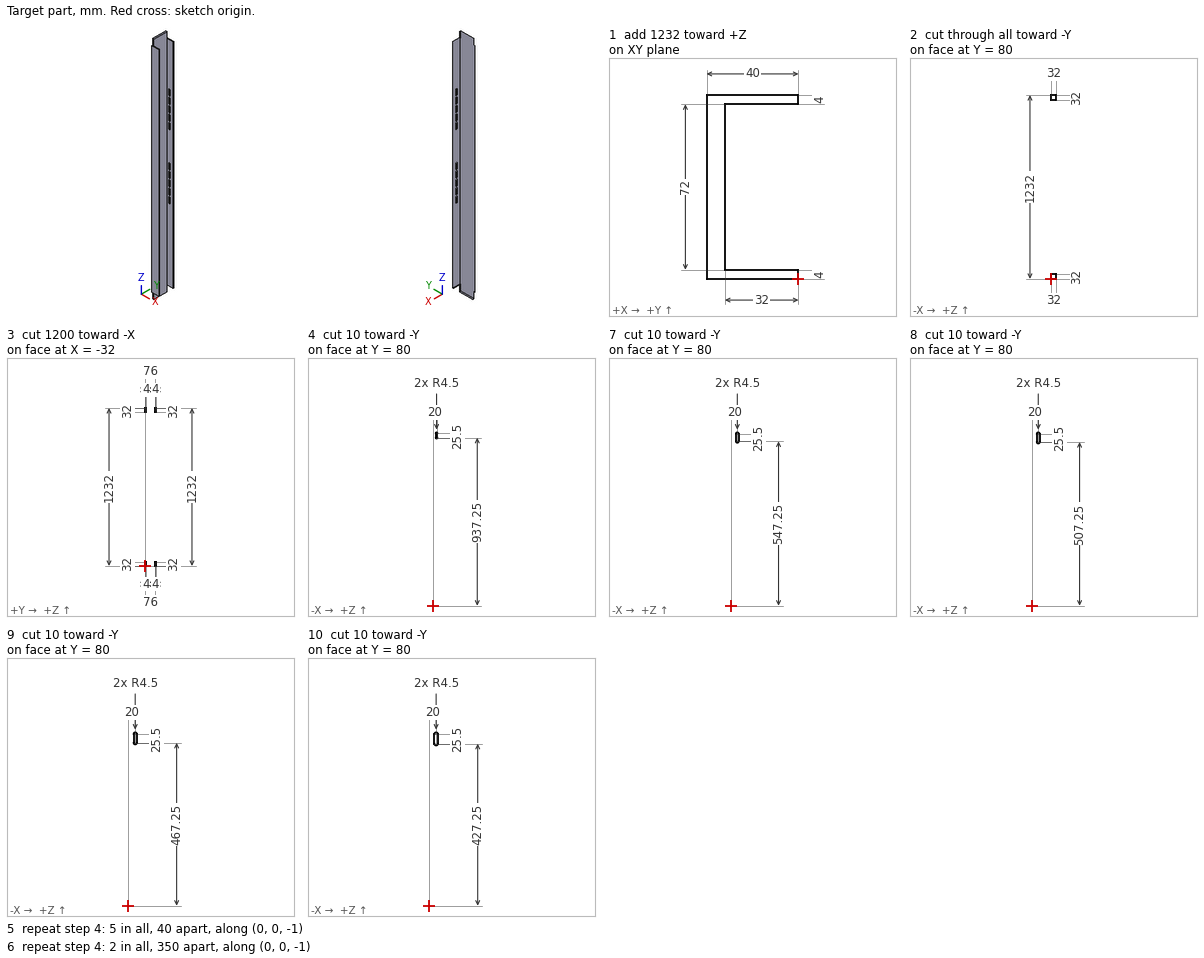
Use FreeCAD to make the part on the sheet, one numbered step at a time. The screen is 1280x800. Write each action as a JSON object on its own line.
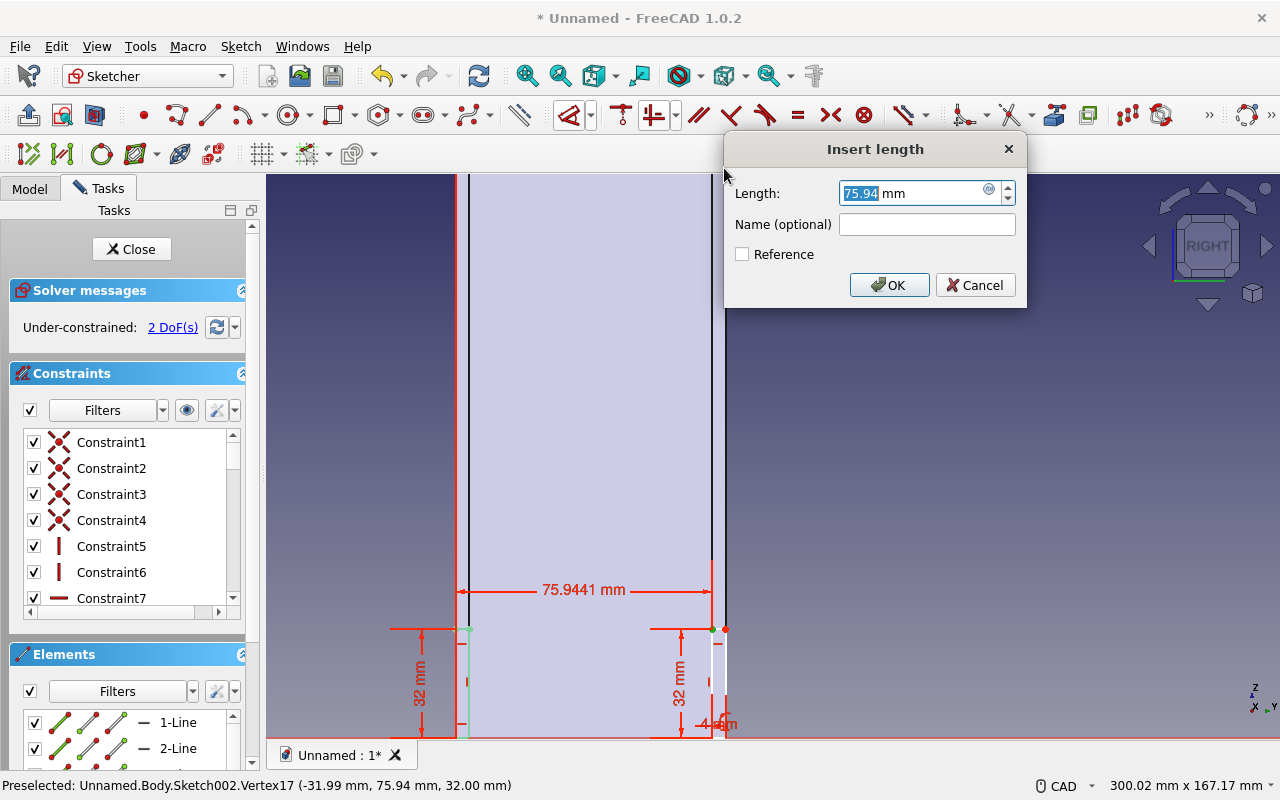
{"action": "type", "text": "76"}
{"action": "key", "text": "Return"}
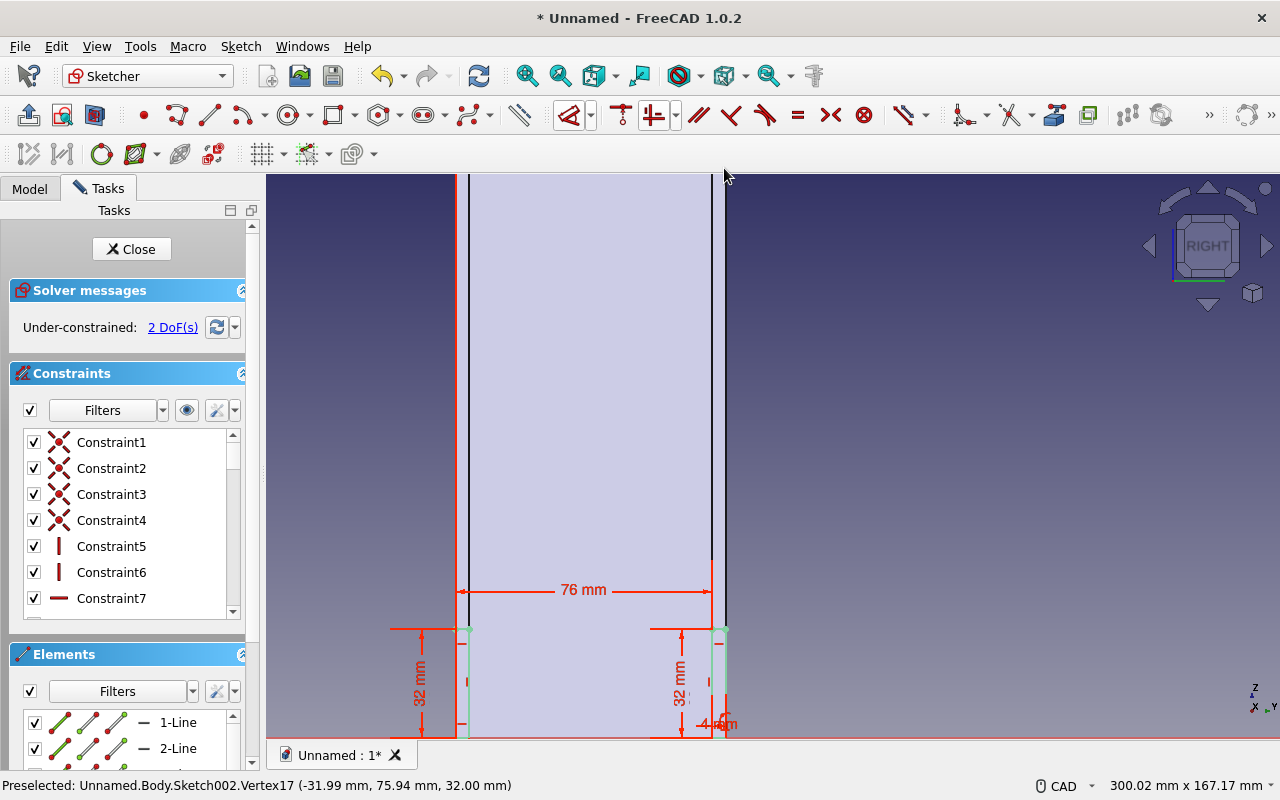
{"action": "scroll", "coordinate": [716, 636], "scroll_direction": "down", "scroll_amount": 12}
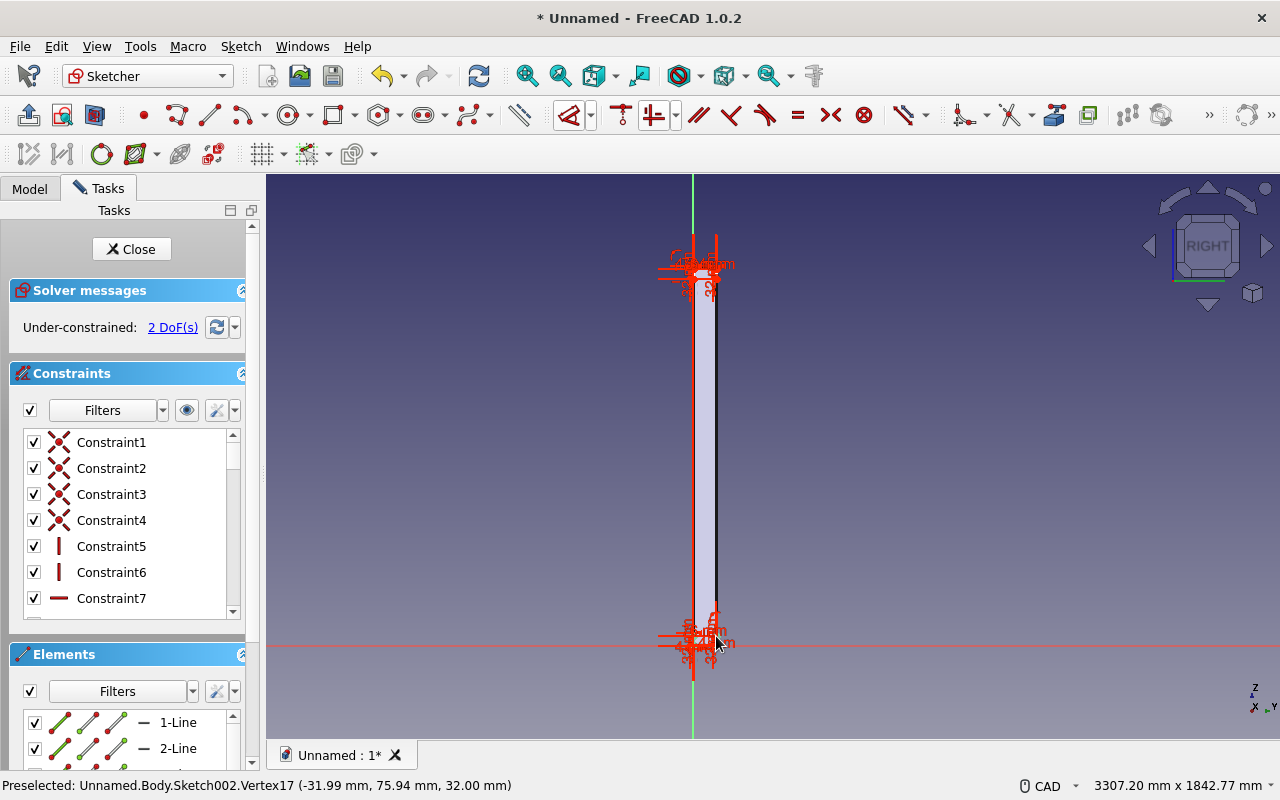
{"action": "scroll", "coordinate": [716, 269], "scroll_direction": "up", "scroll_amount": 12}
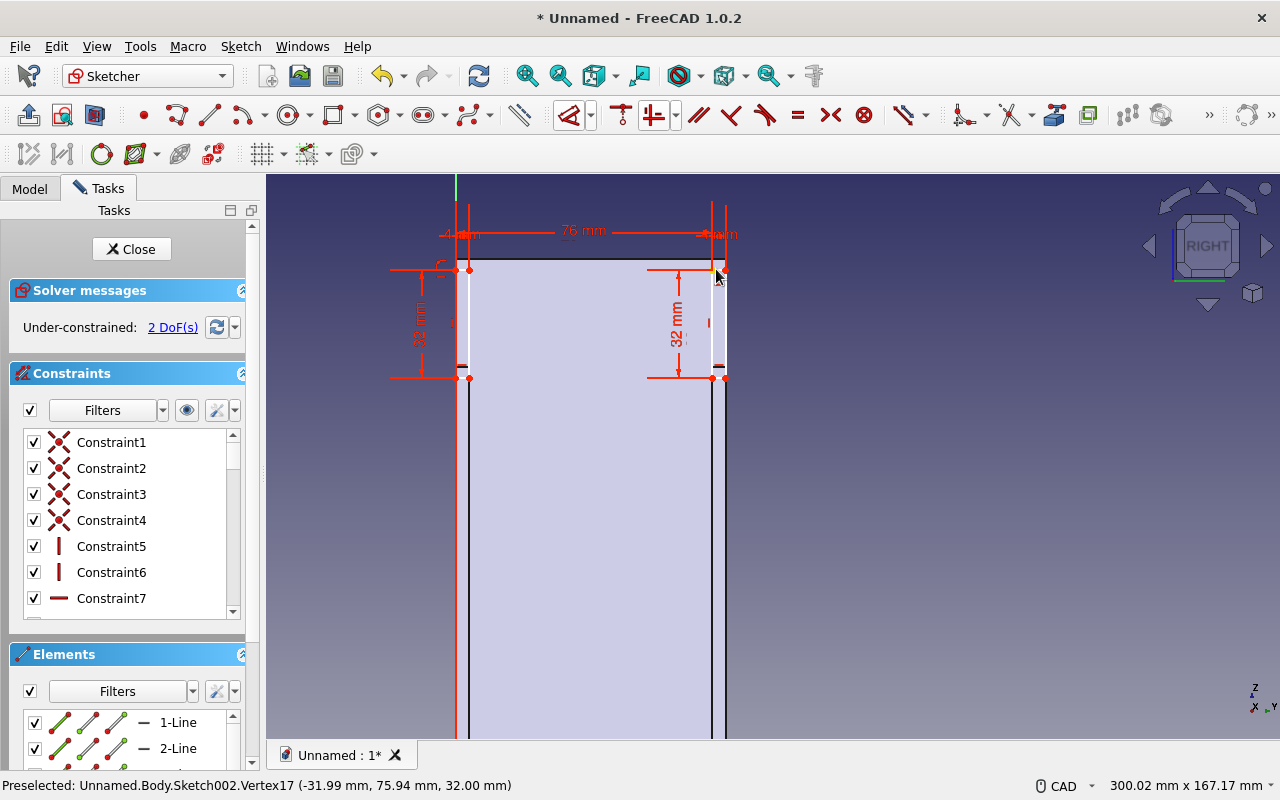
{"action": "left_click", "coordinate": [712, 270]}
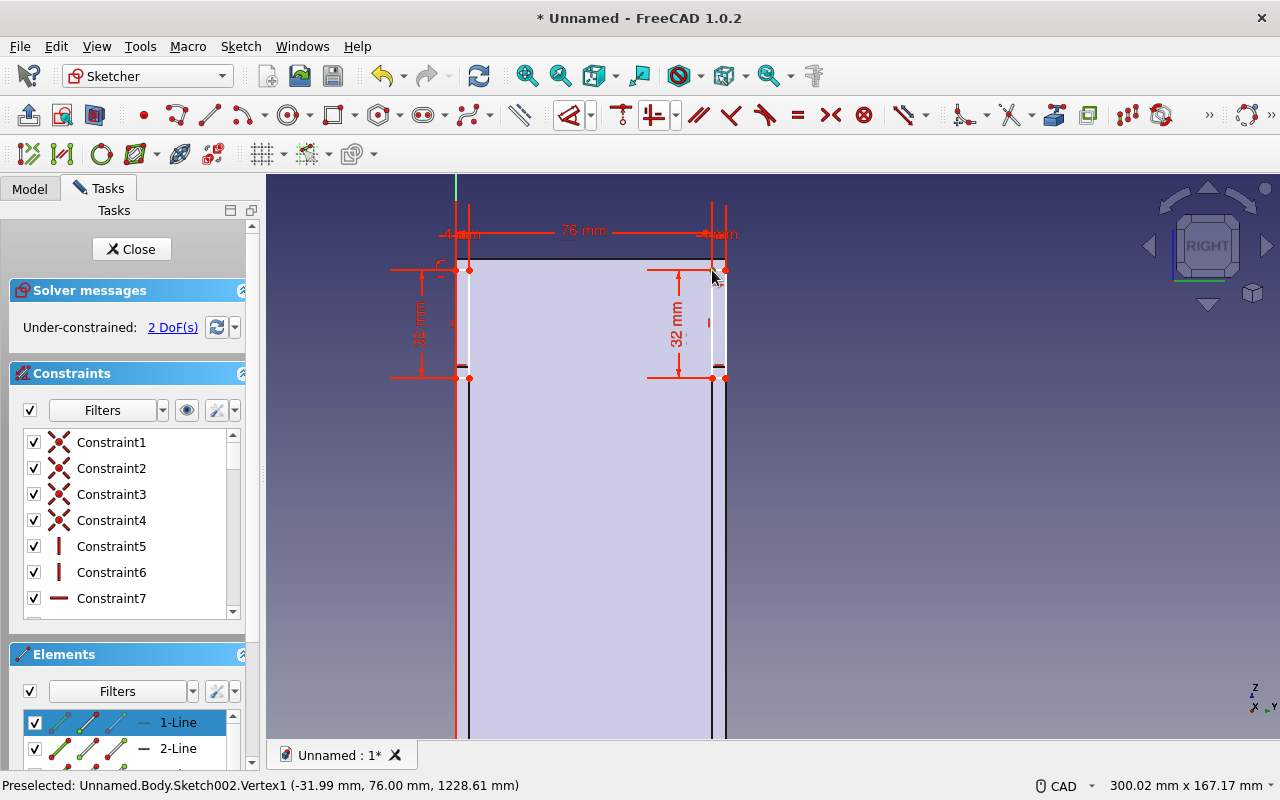
{"action": "left_click", "coordinate": [590, 116]}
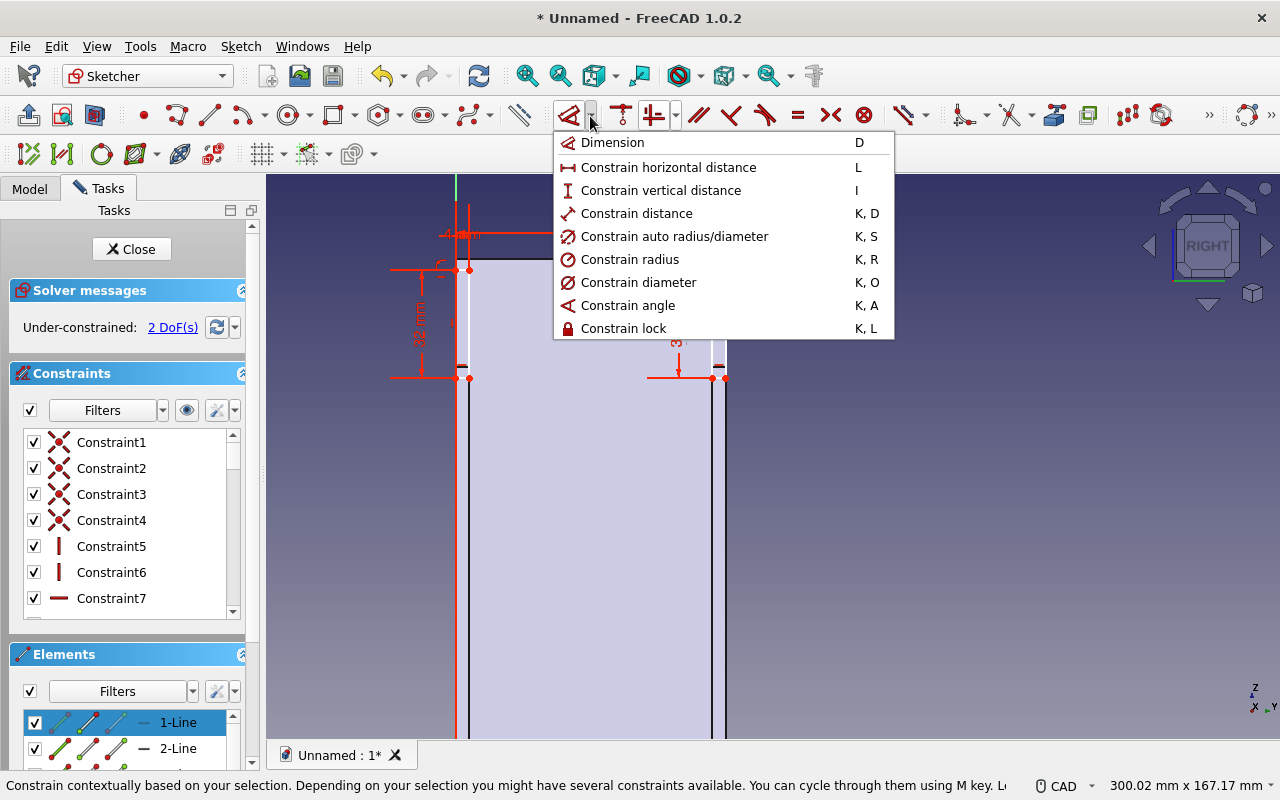
{"action": "left_click", "coordinate": [724, 190]}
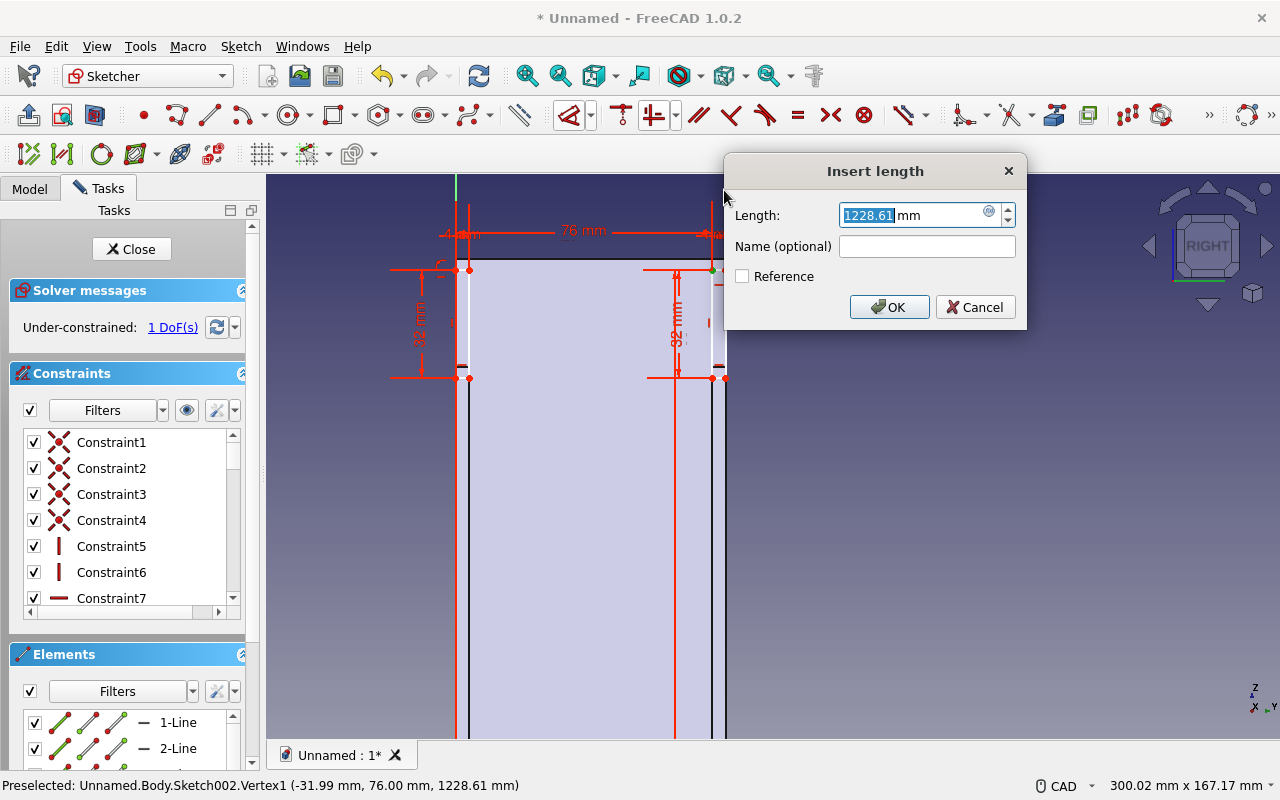
{"action": "type", "text": "1232"}
{"action": "key", "text": "Return"}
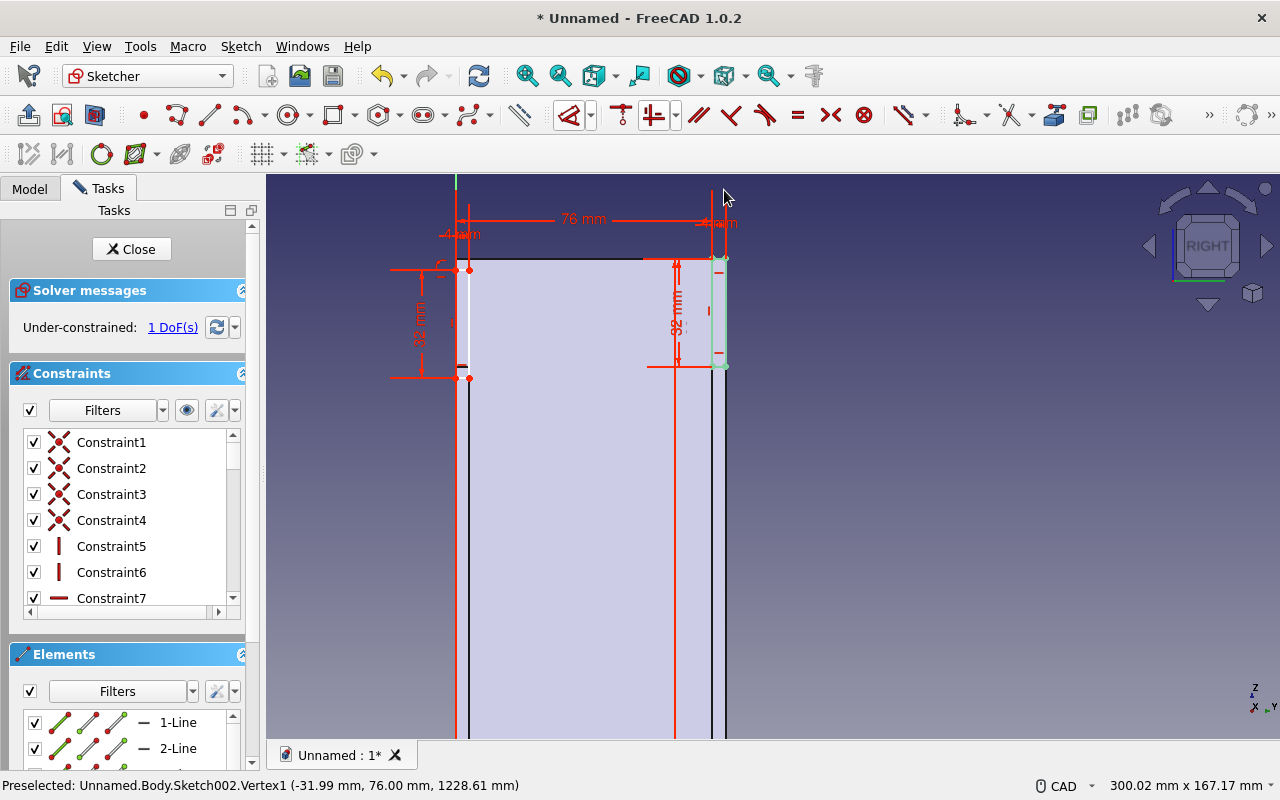
{"action": "left_click", "coordinate": [456, 270]}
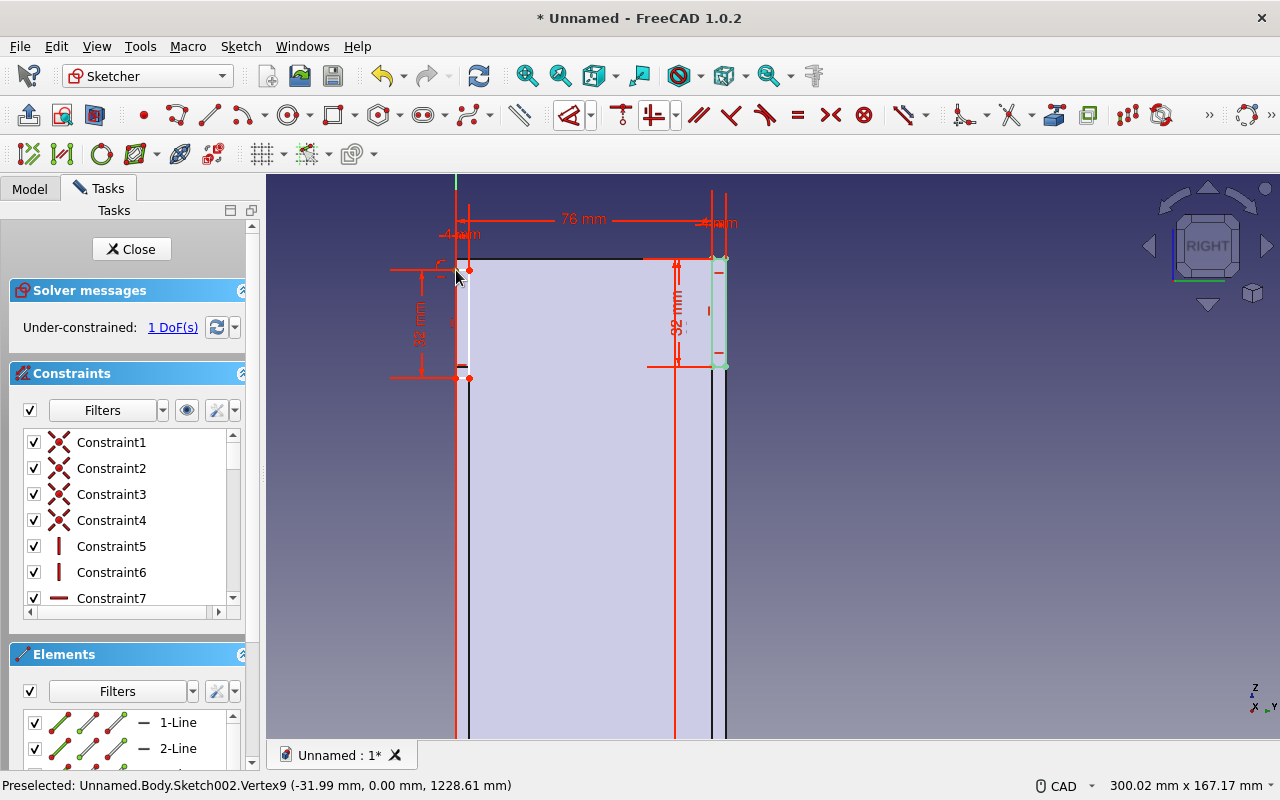
{"action": "left_click", "coordinate": [590, 116]}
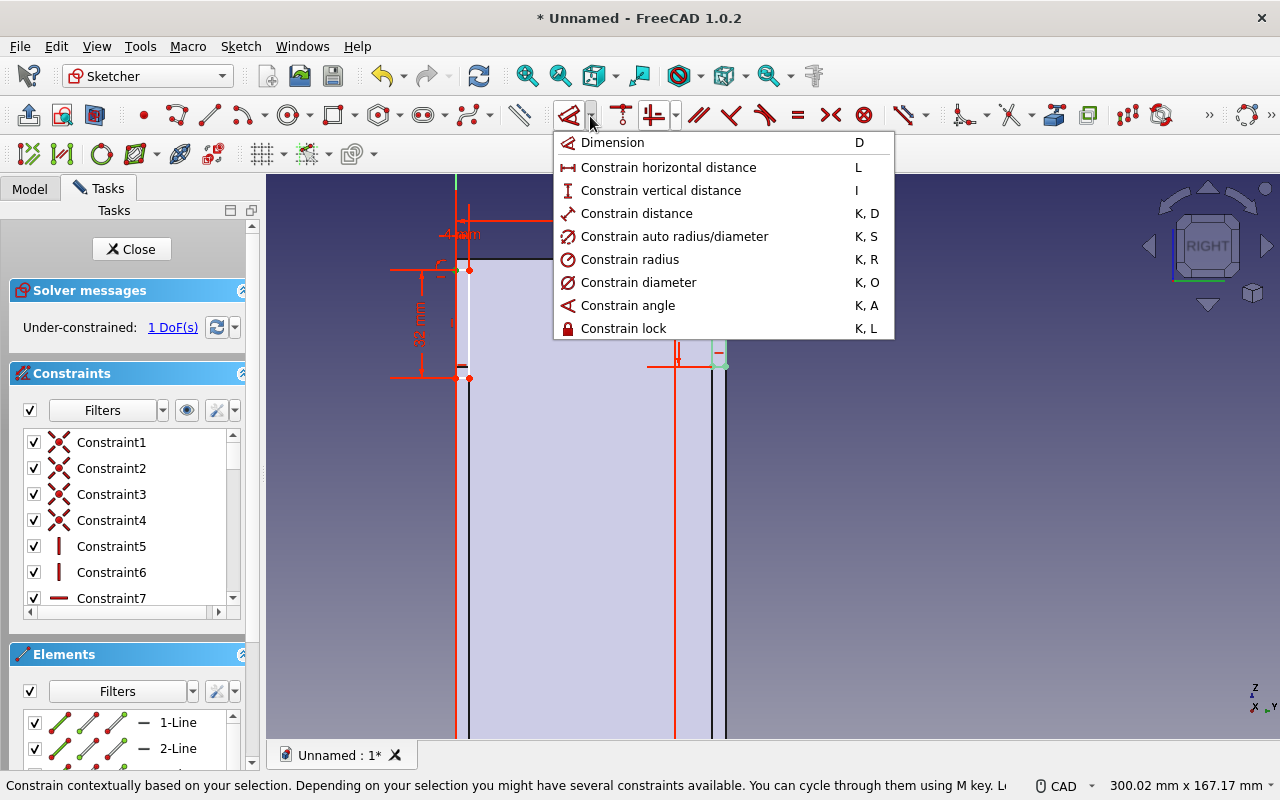
{"action": "left_click", "coordinate": [724, 190]}